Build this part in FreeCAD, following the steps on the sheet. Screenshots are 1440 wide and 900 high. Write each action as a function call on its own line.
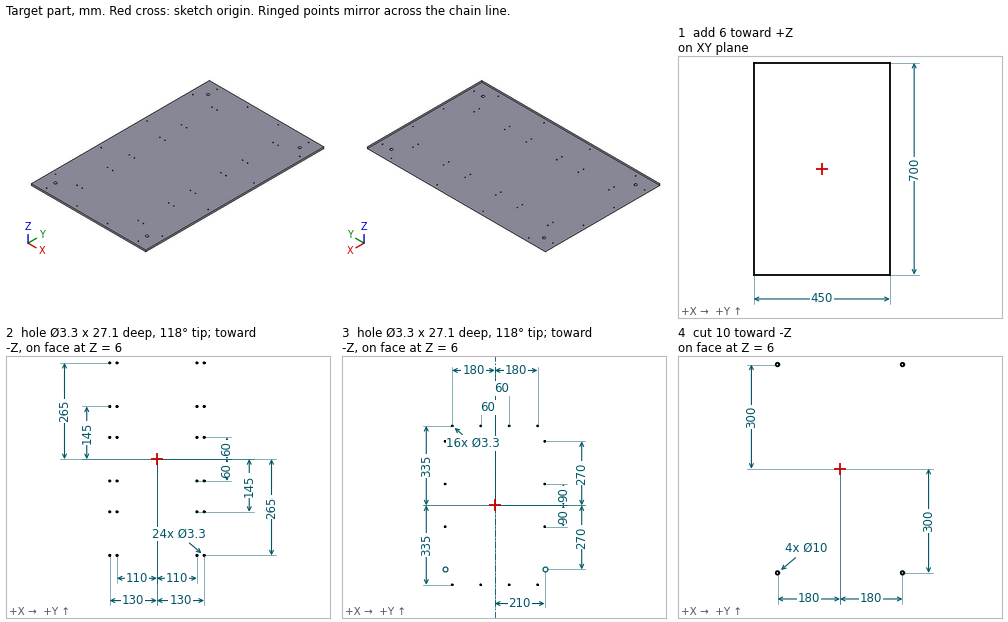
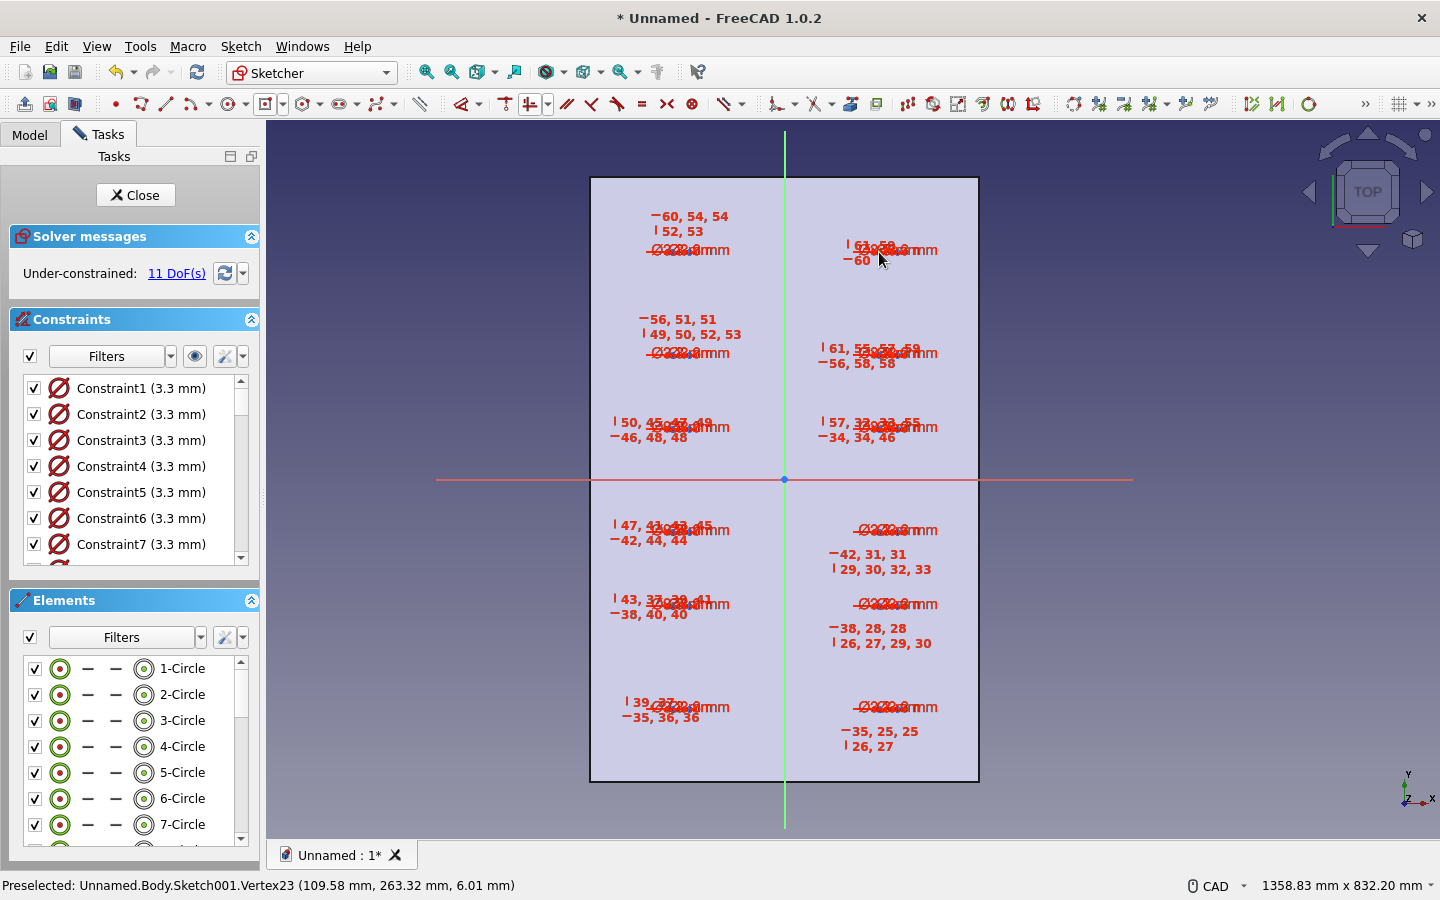
click(897, 252)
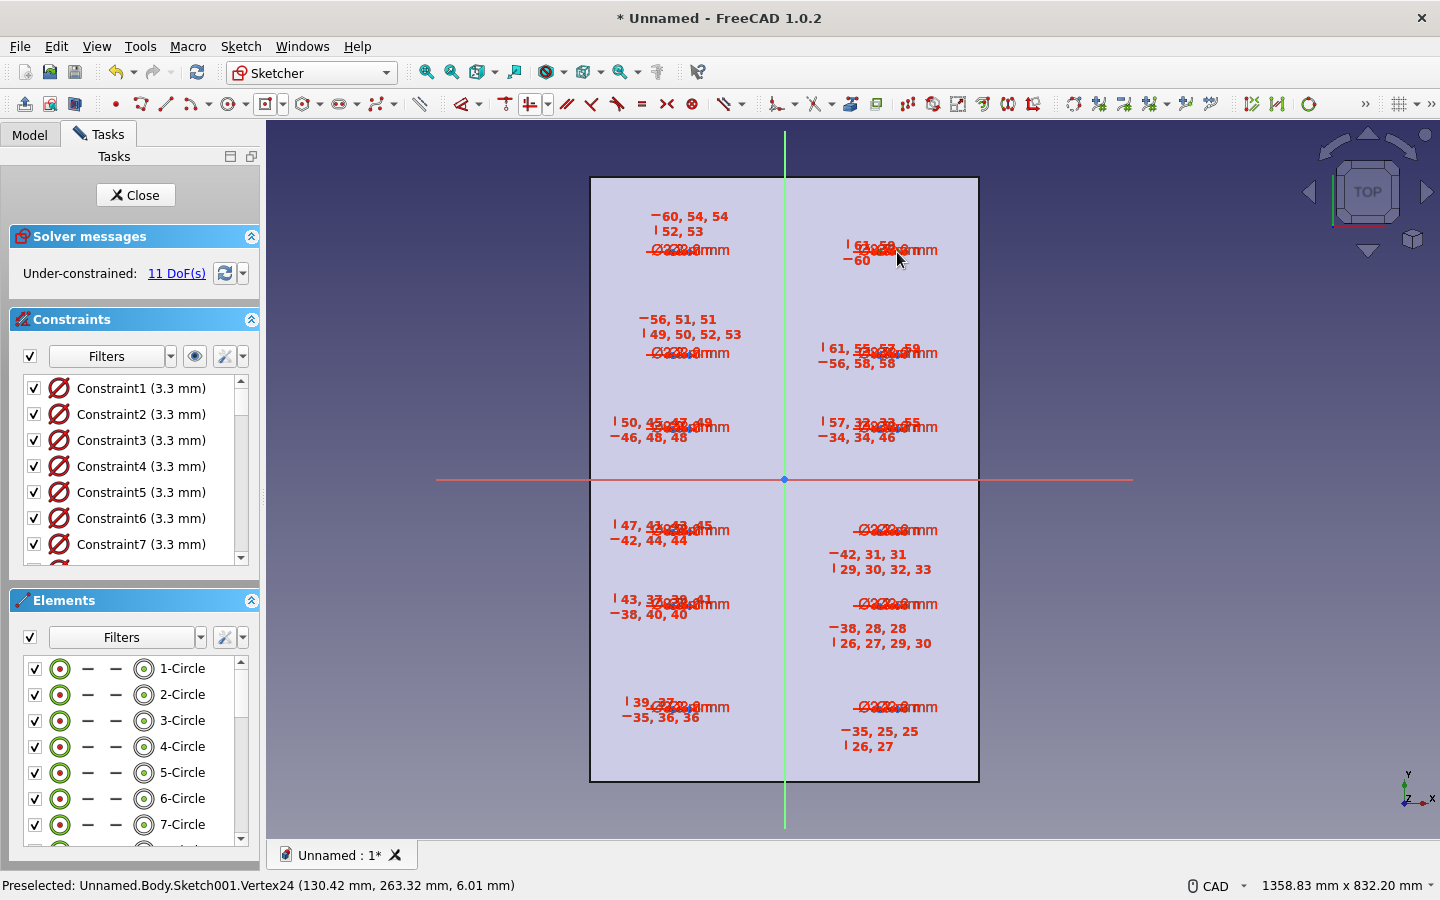
click(548, 104)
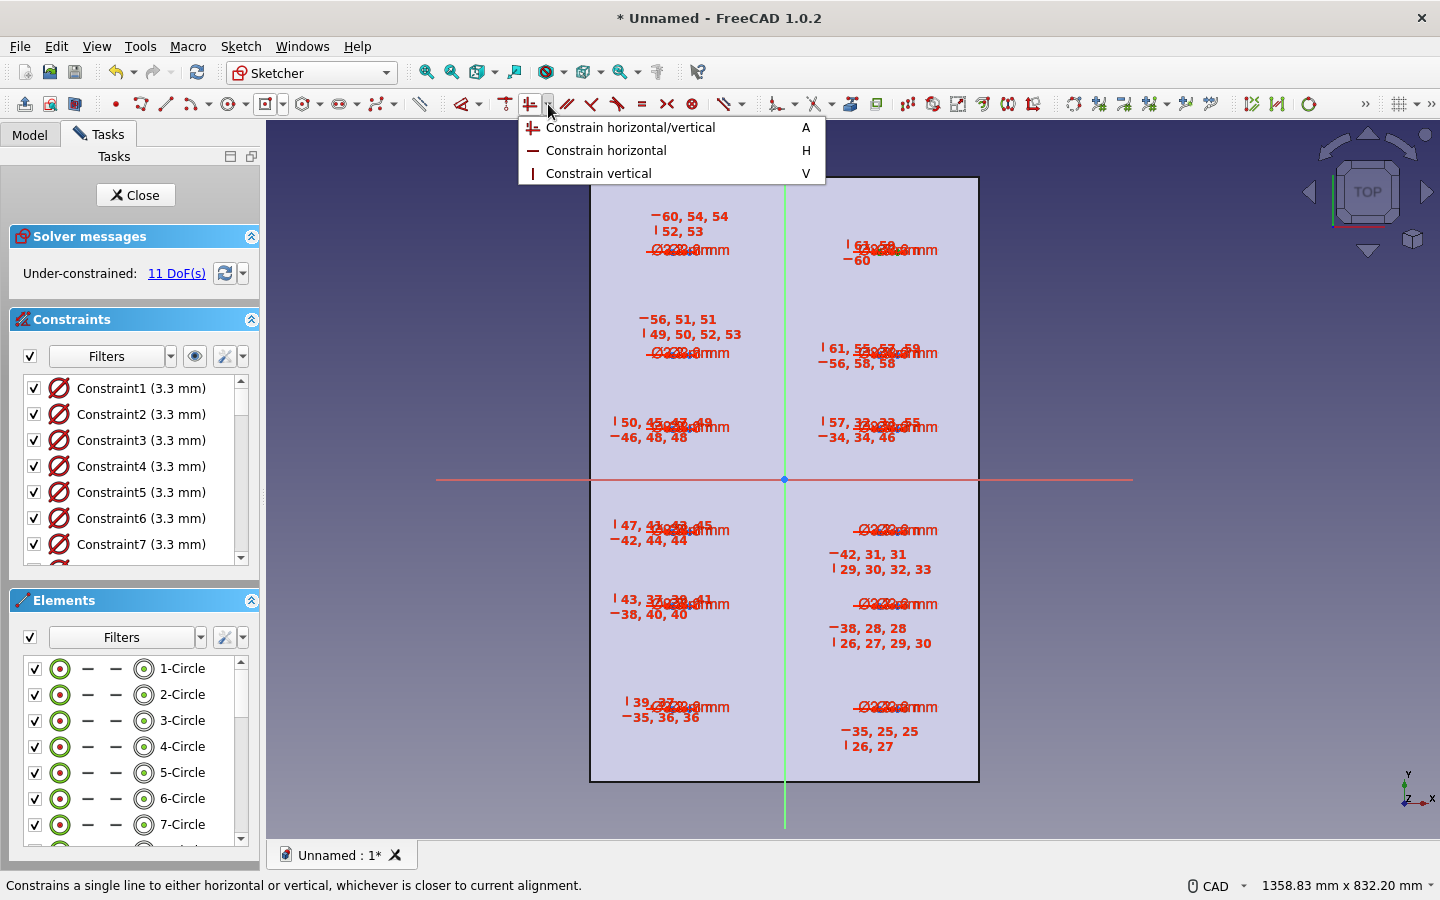
click(672, 150)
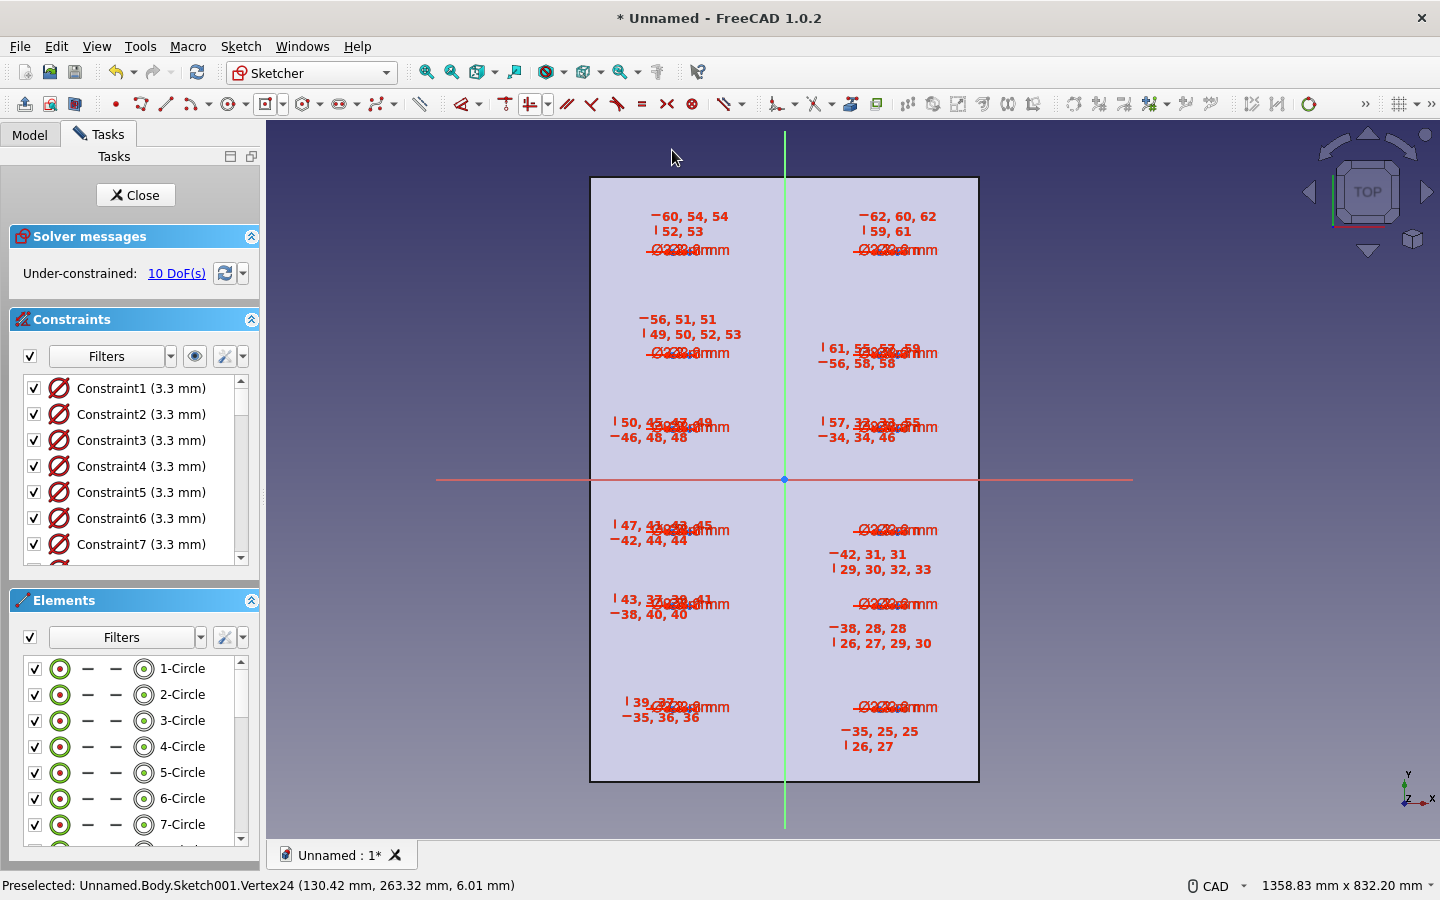
click(879, 532)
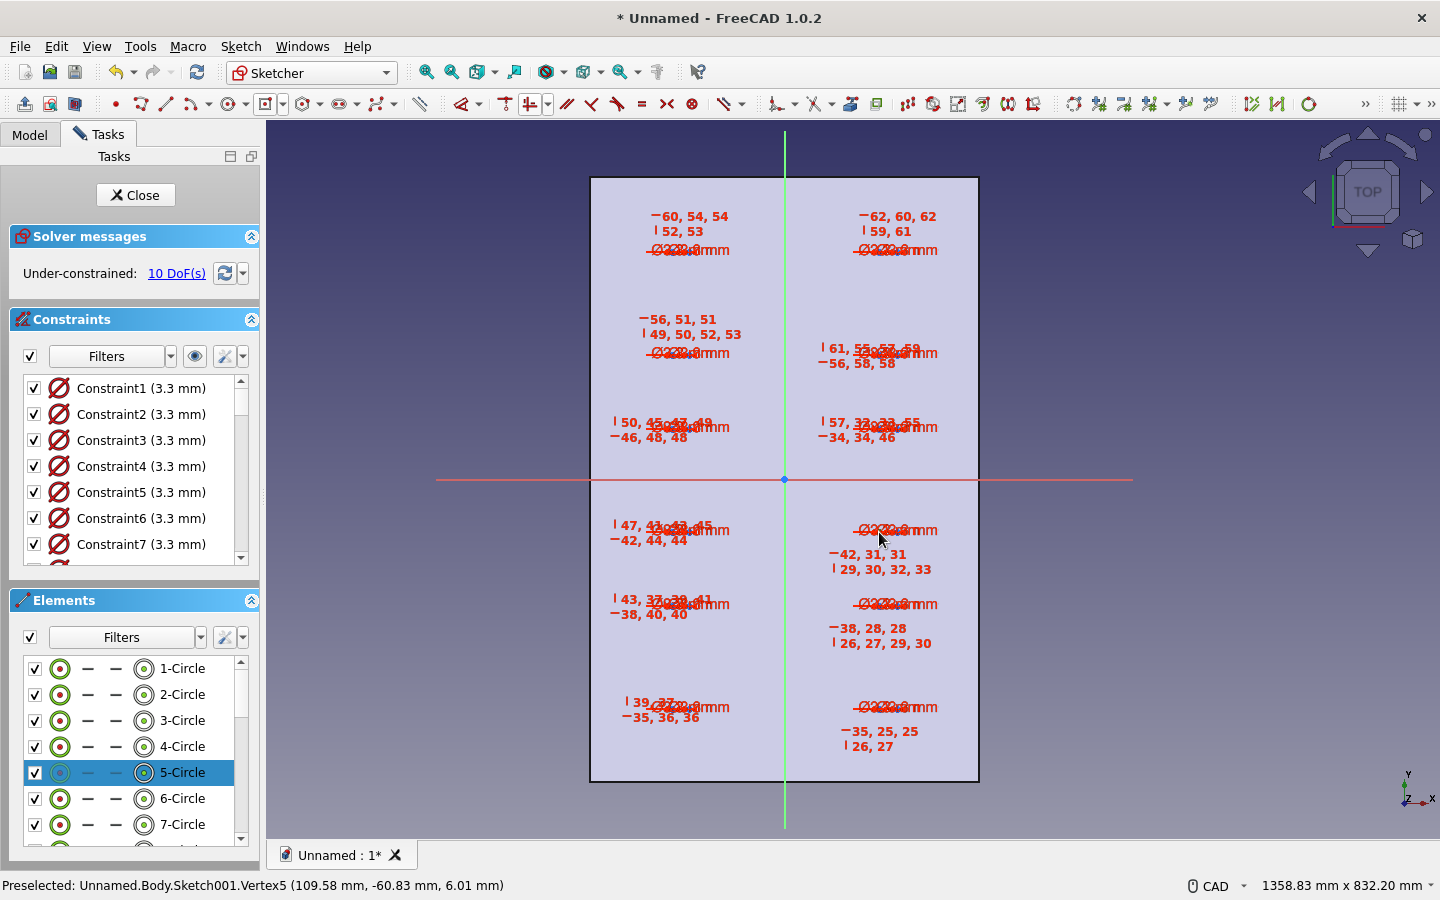
click(478, 104)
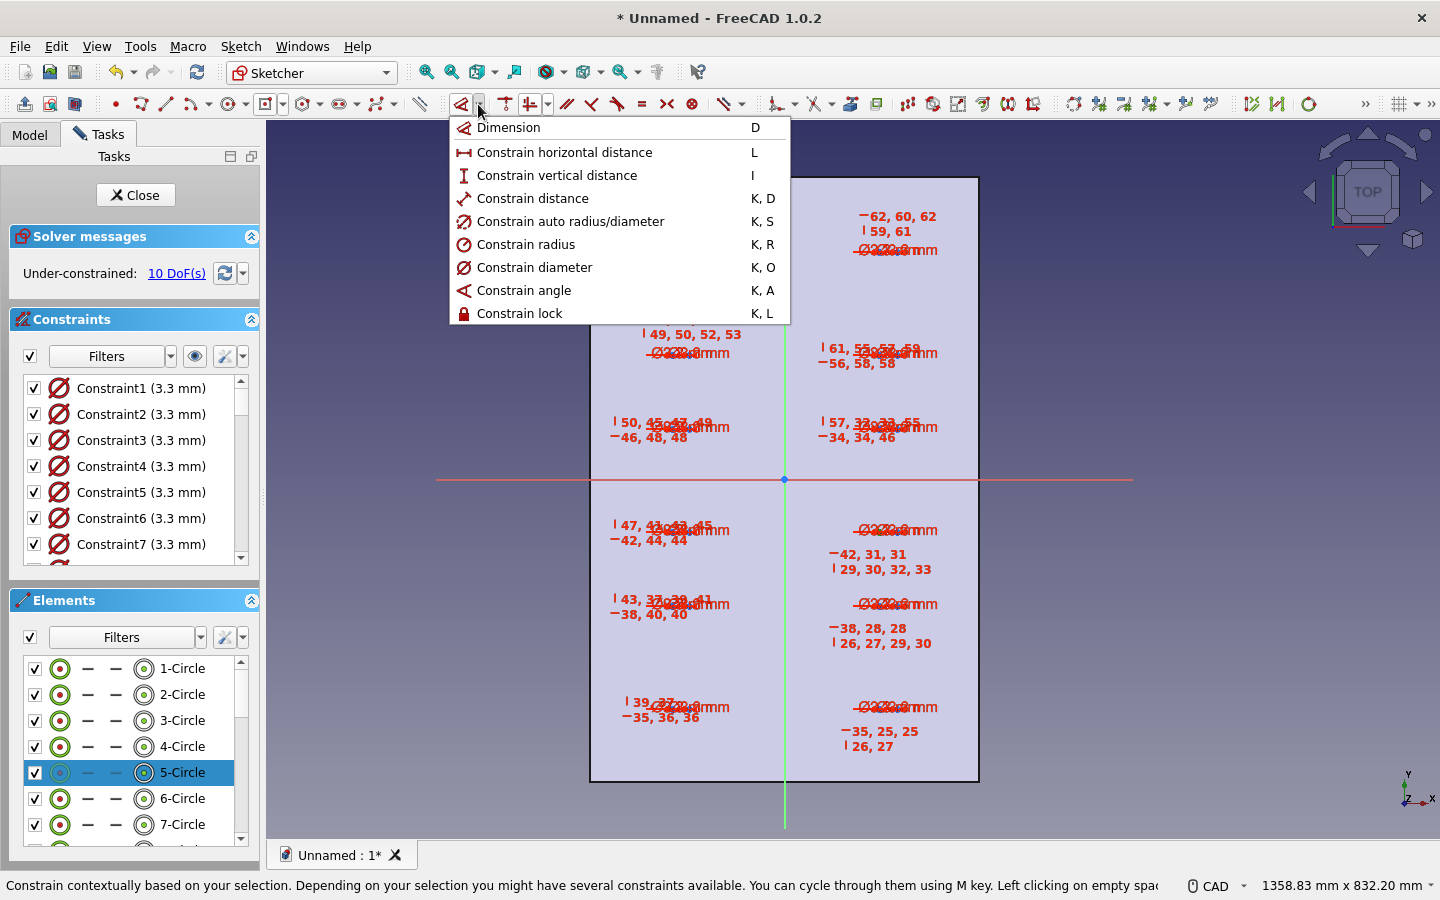
click(620, 176)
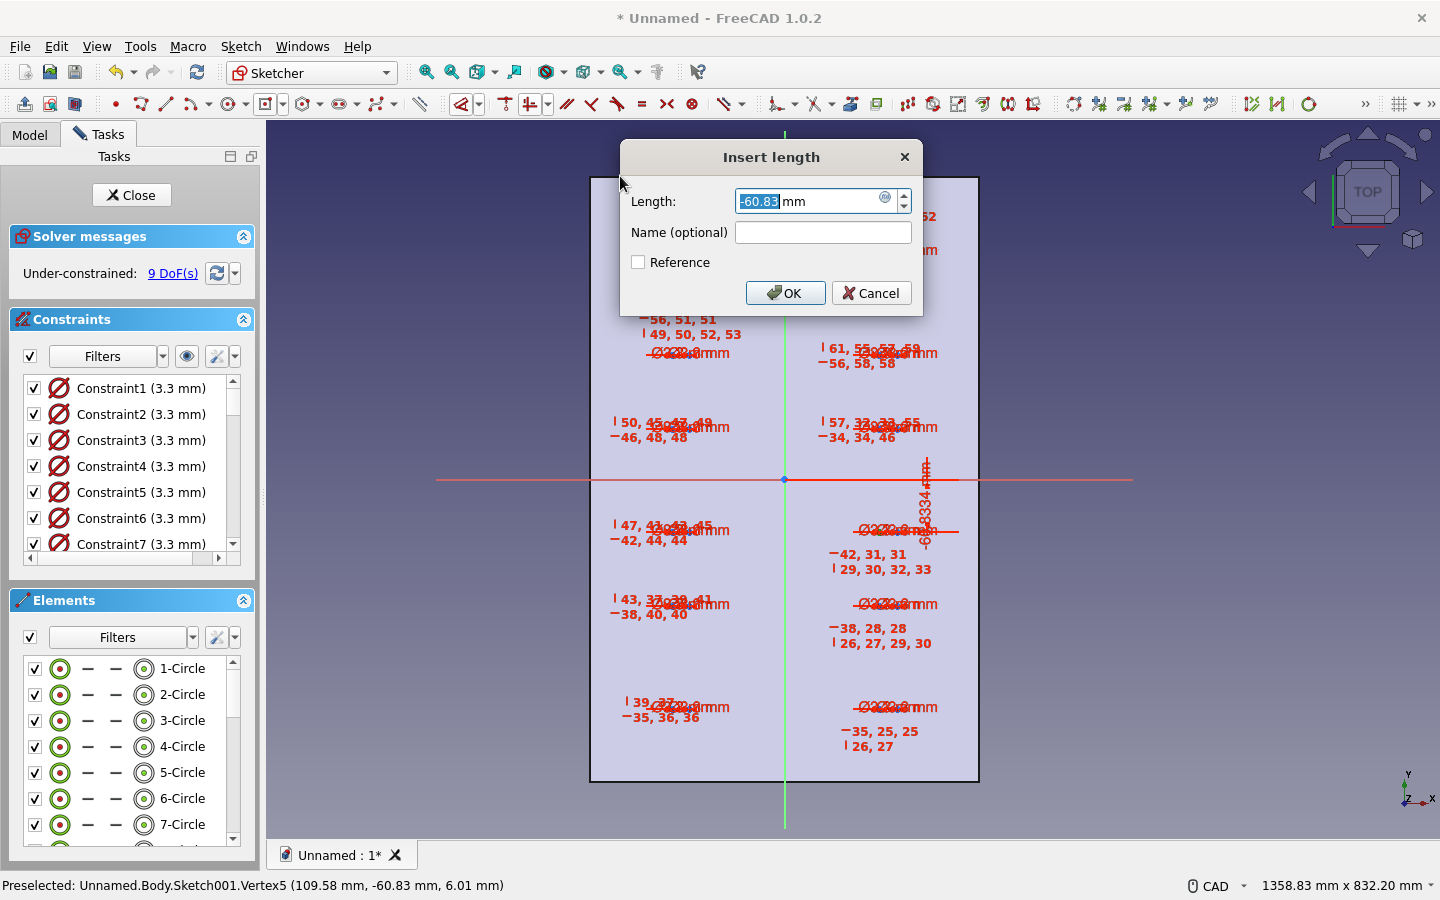
text(-60)
key(Return)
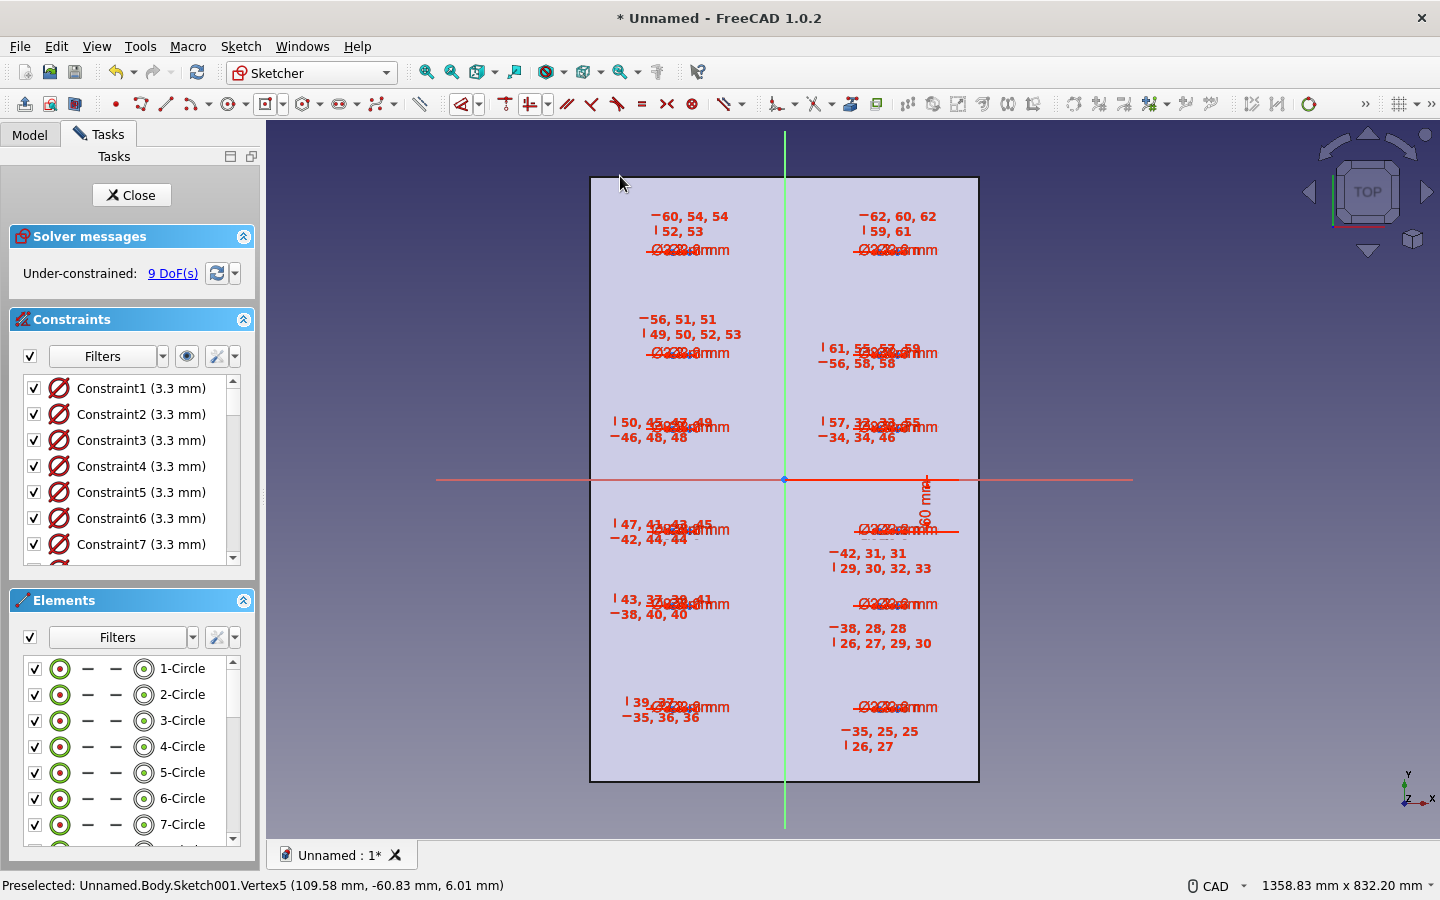
click(897, 429)